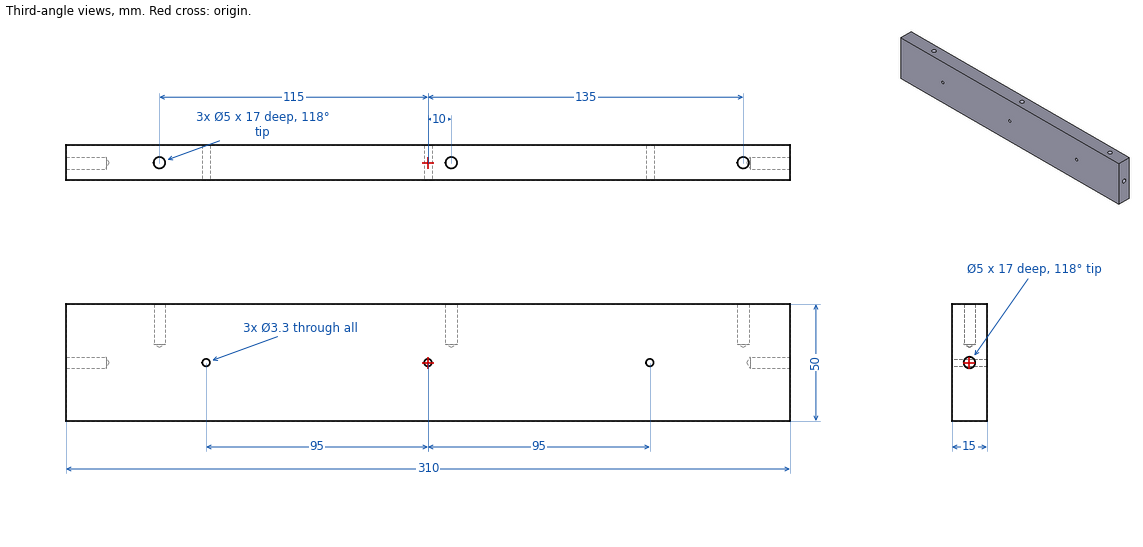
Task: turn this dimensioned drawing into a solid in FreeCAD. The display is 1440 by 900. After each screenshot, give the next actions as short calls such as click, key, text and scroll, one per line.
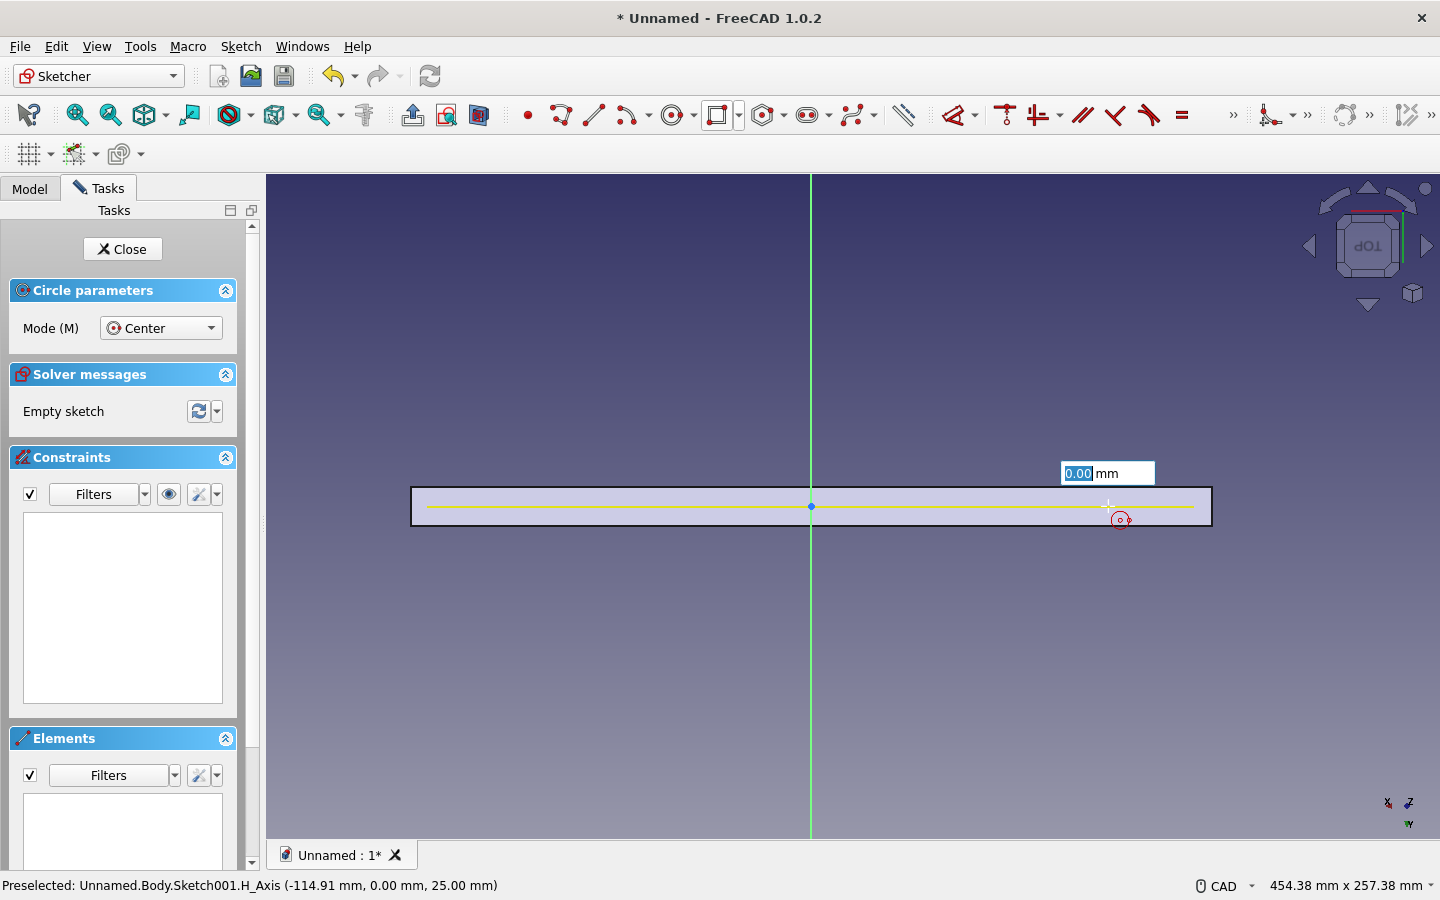
scroll(1106, 513, up, 5)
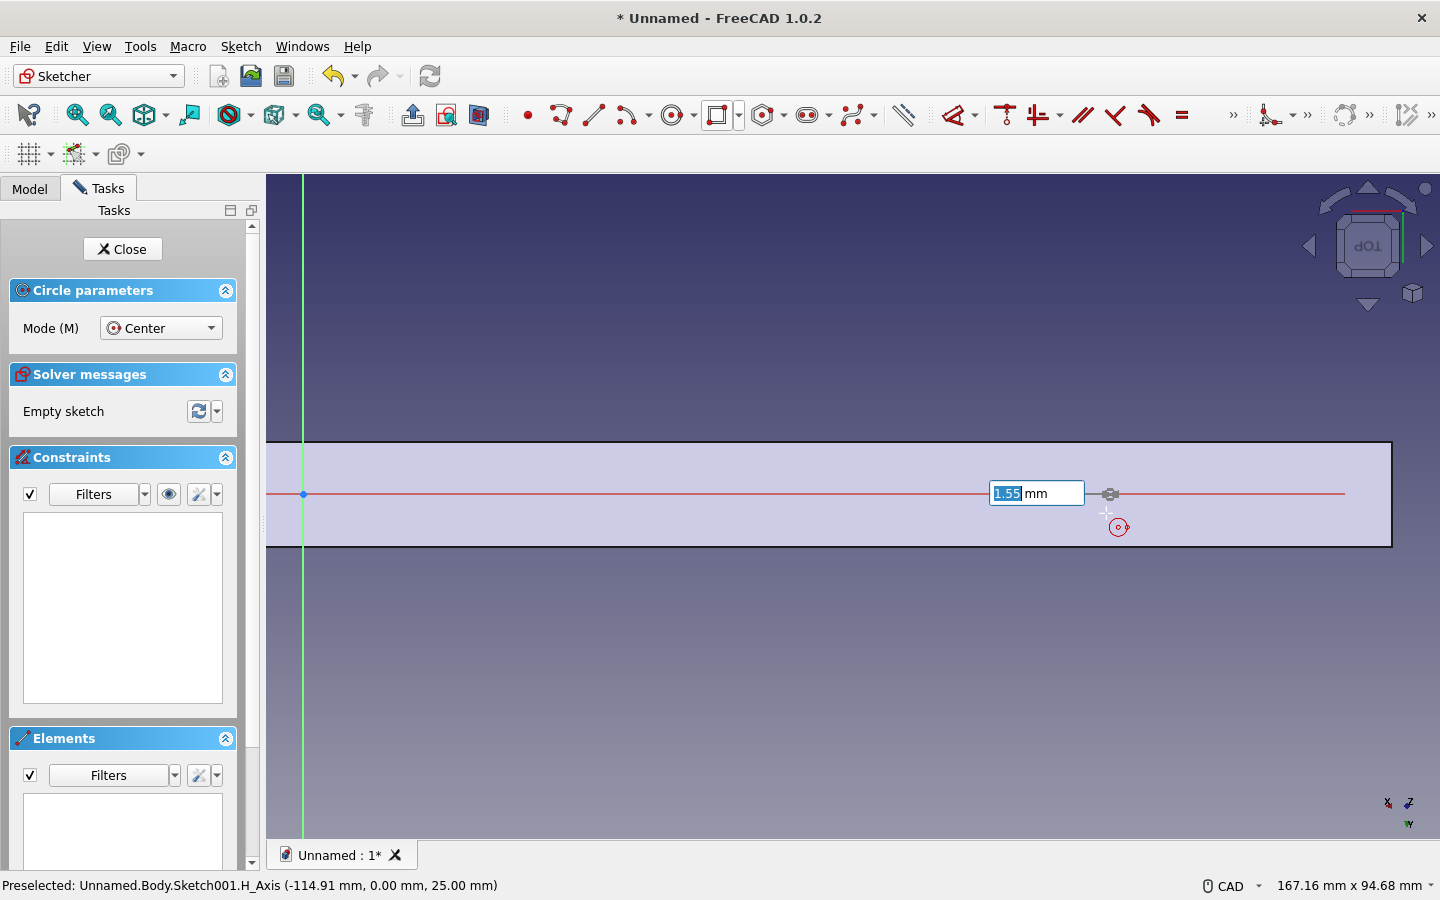
click(1105, 511)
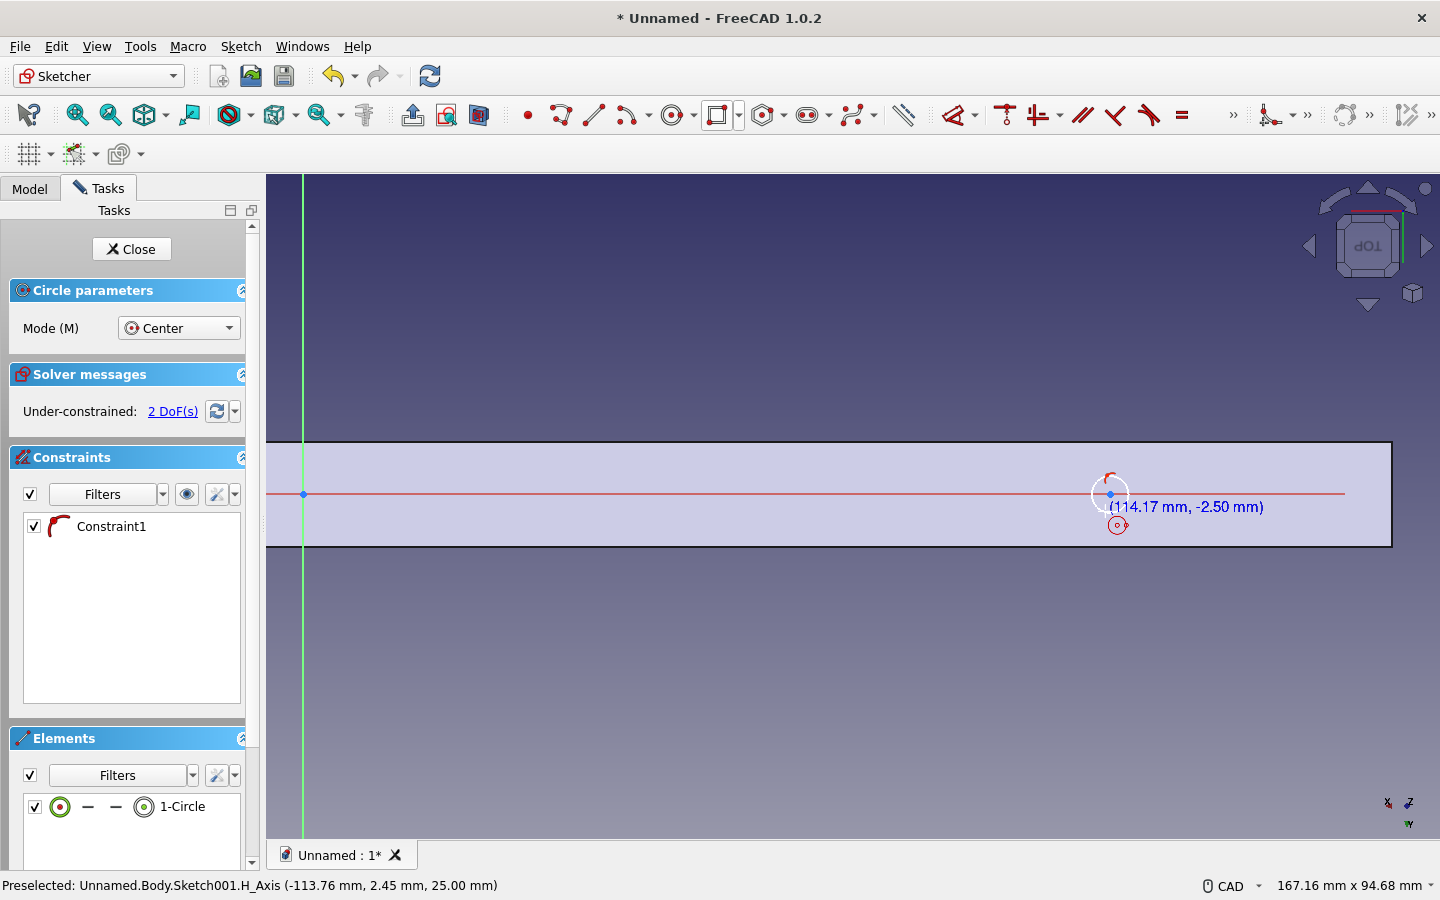
scroll(1105, 514, down, 5)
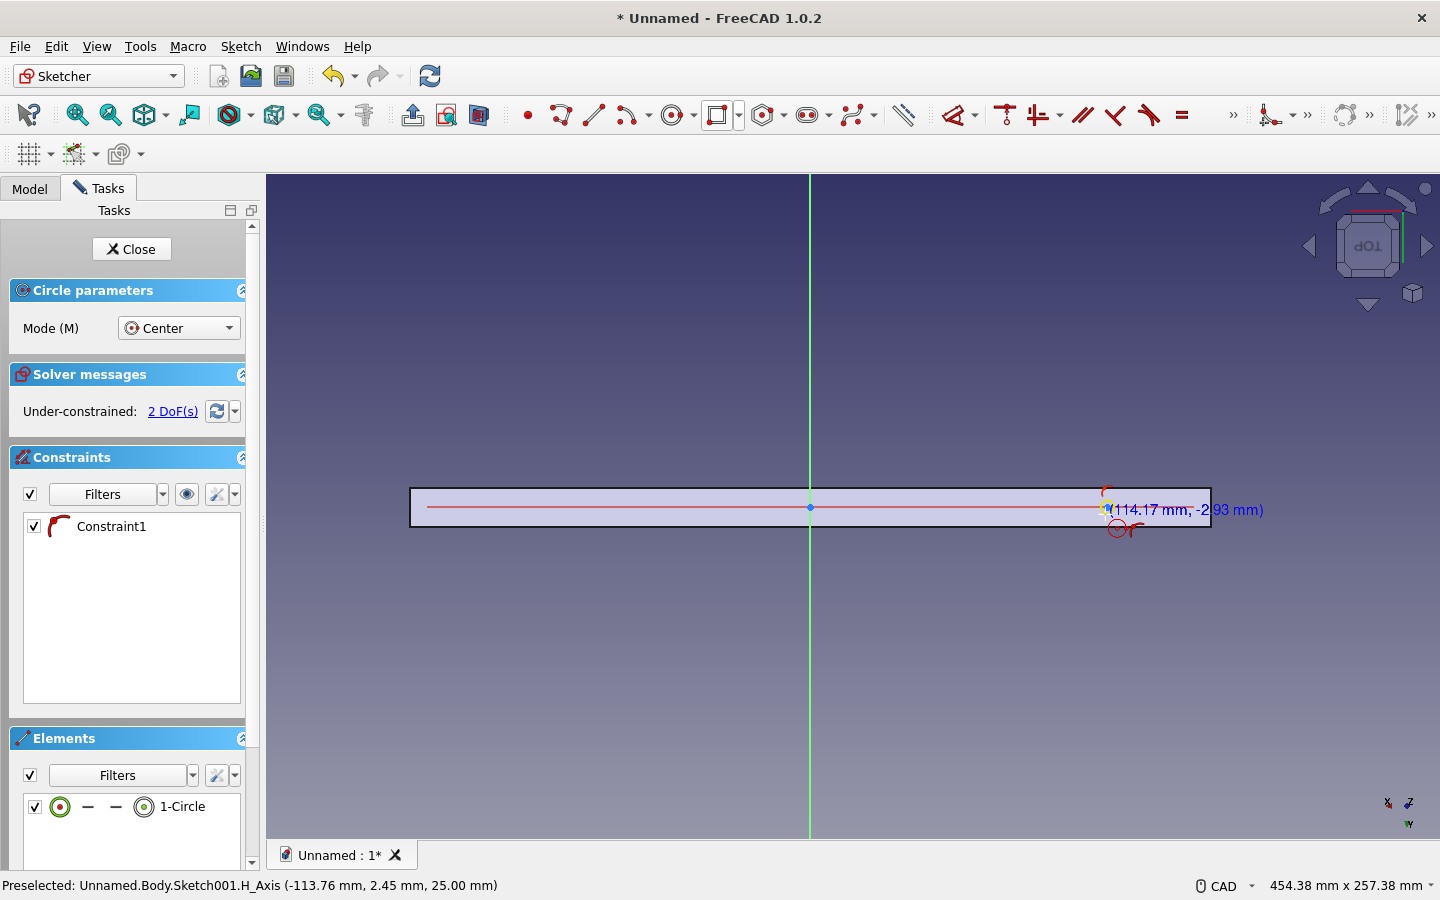
scroll(785, 507, up, 7)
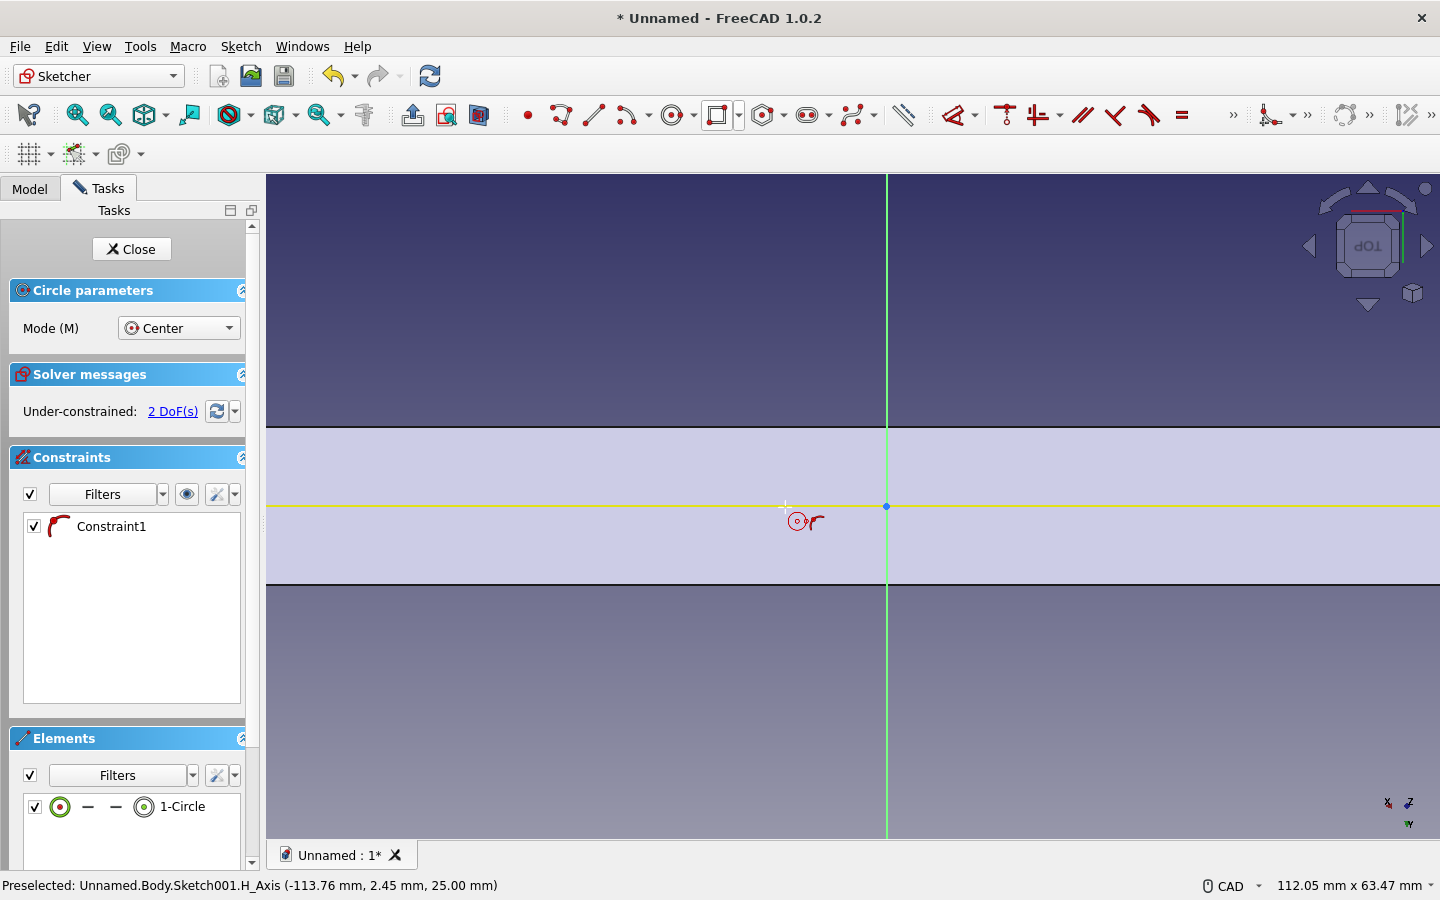
scroll(785, 507, down, 7)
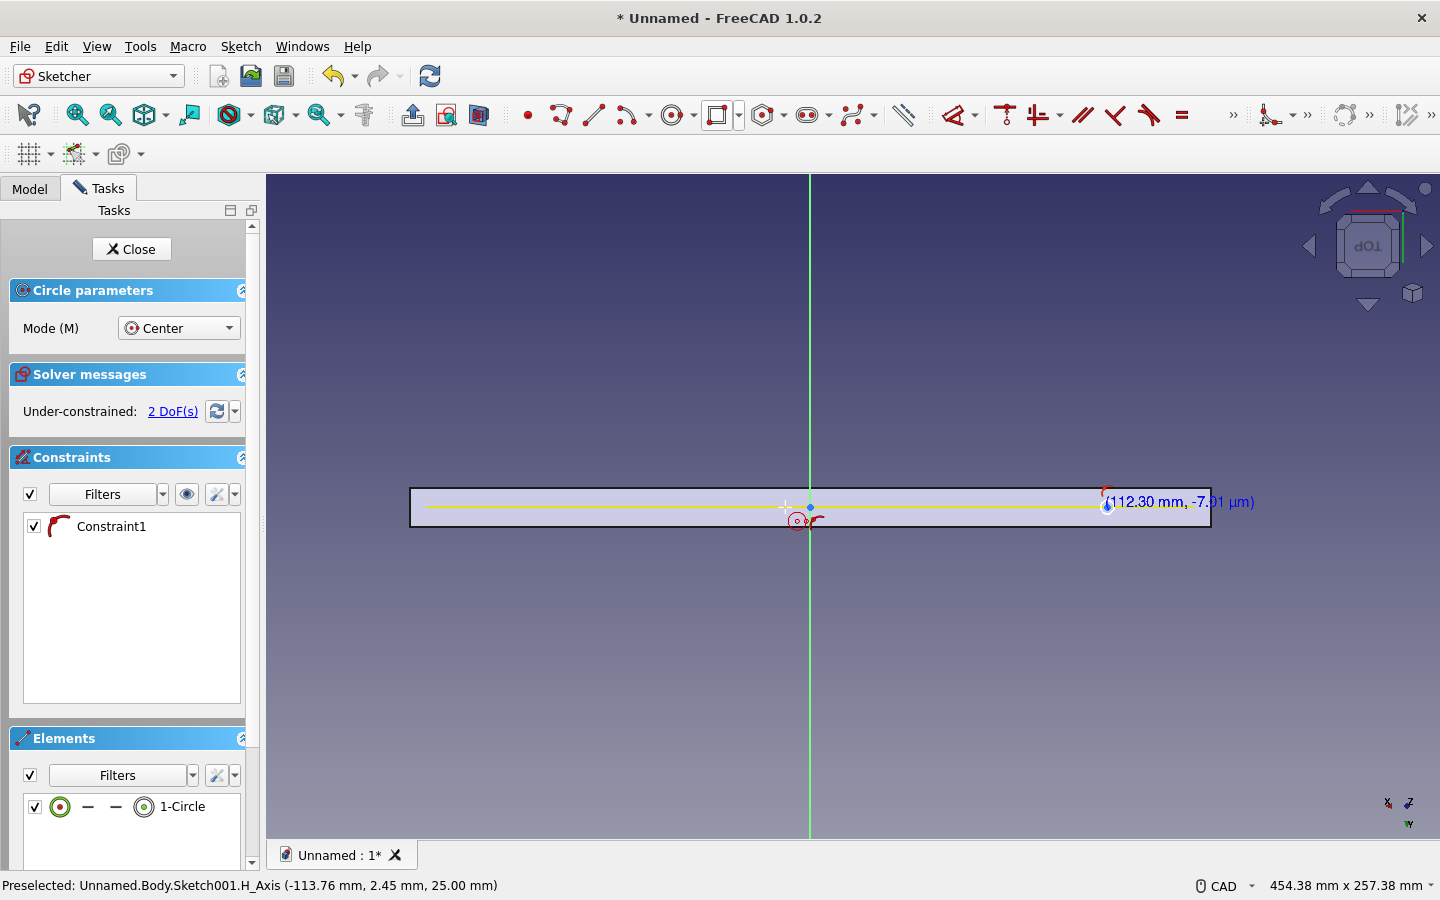
click(785, 507)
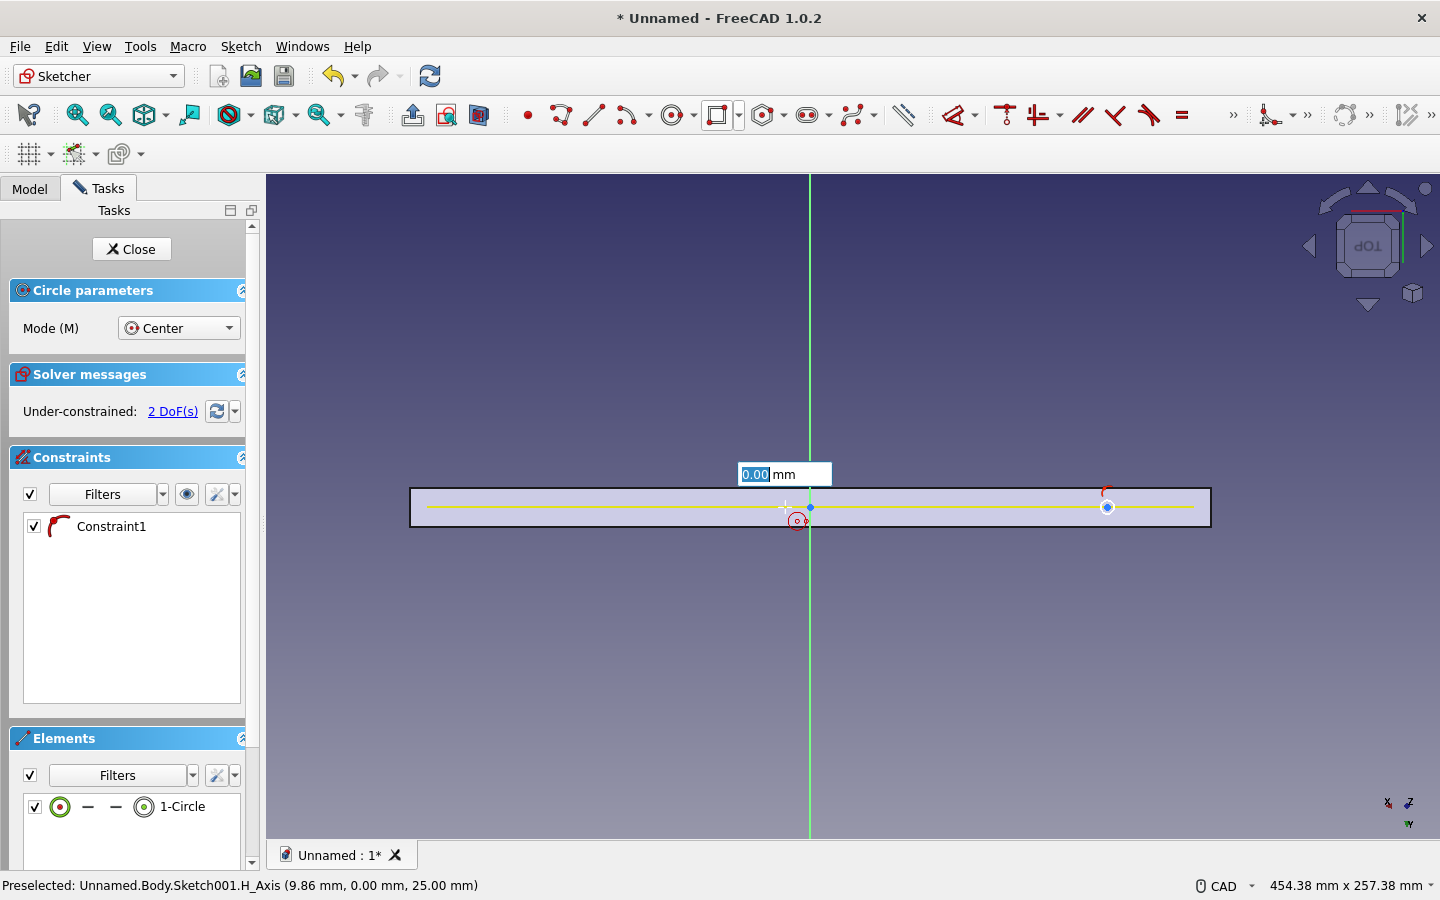
scroll(782, 513, up, 5)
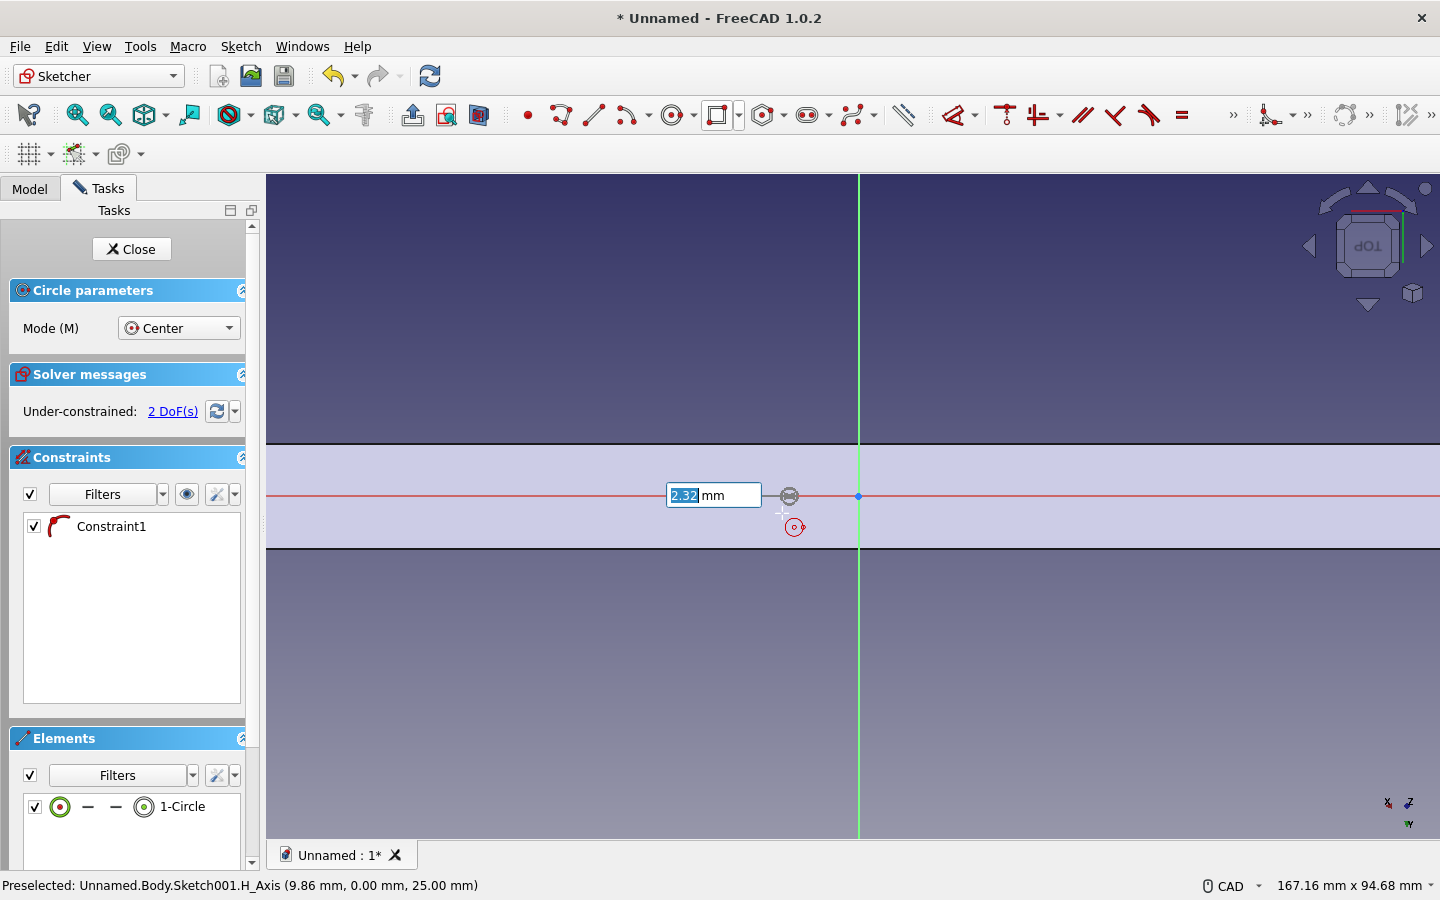
click(782, 513)